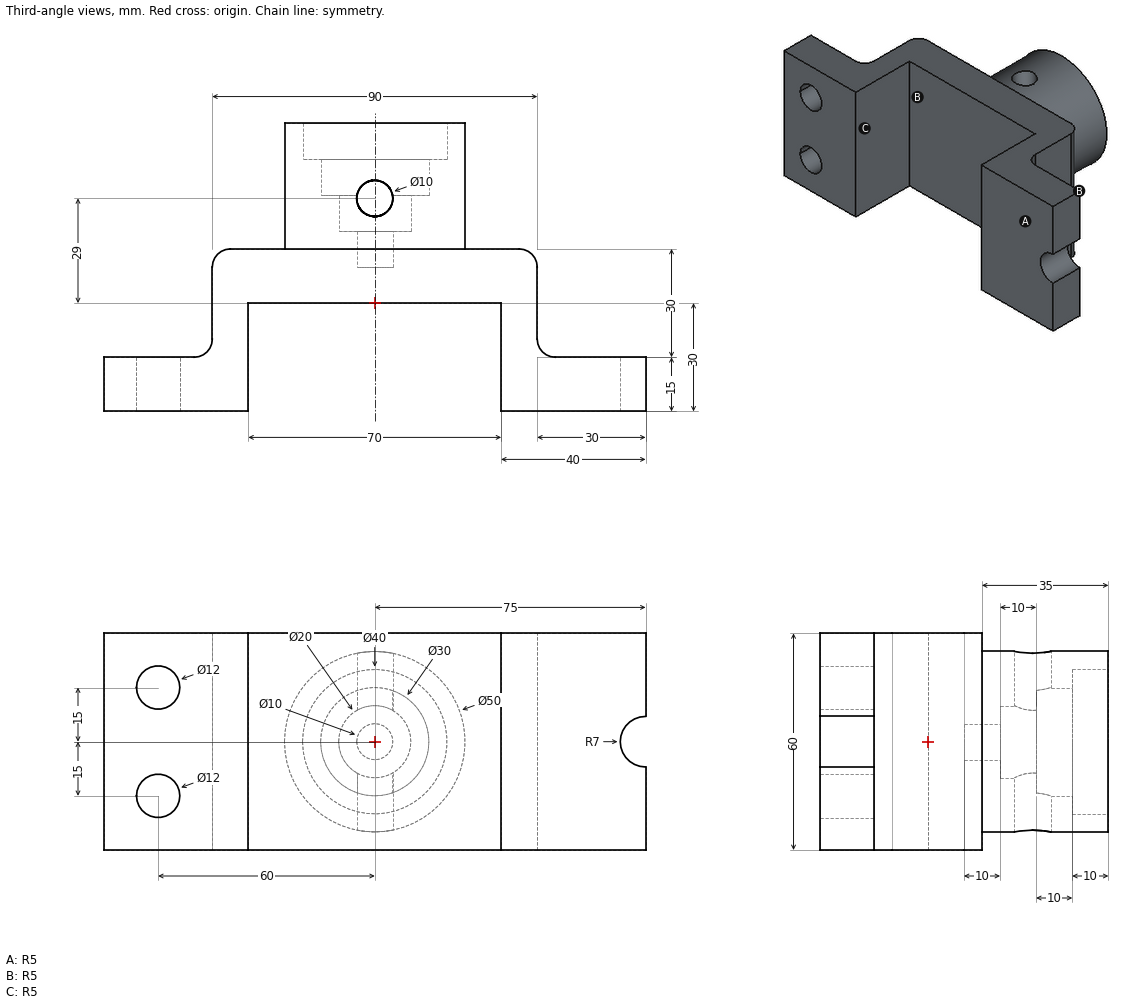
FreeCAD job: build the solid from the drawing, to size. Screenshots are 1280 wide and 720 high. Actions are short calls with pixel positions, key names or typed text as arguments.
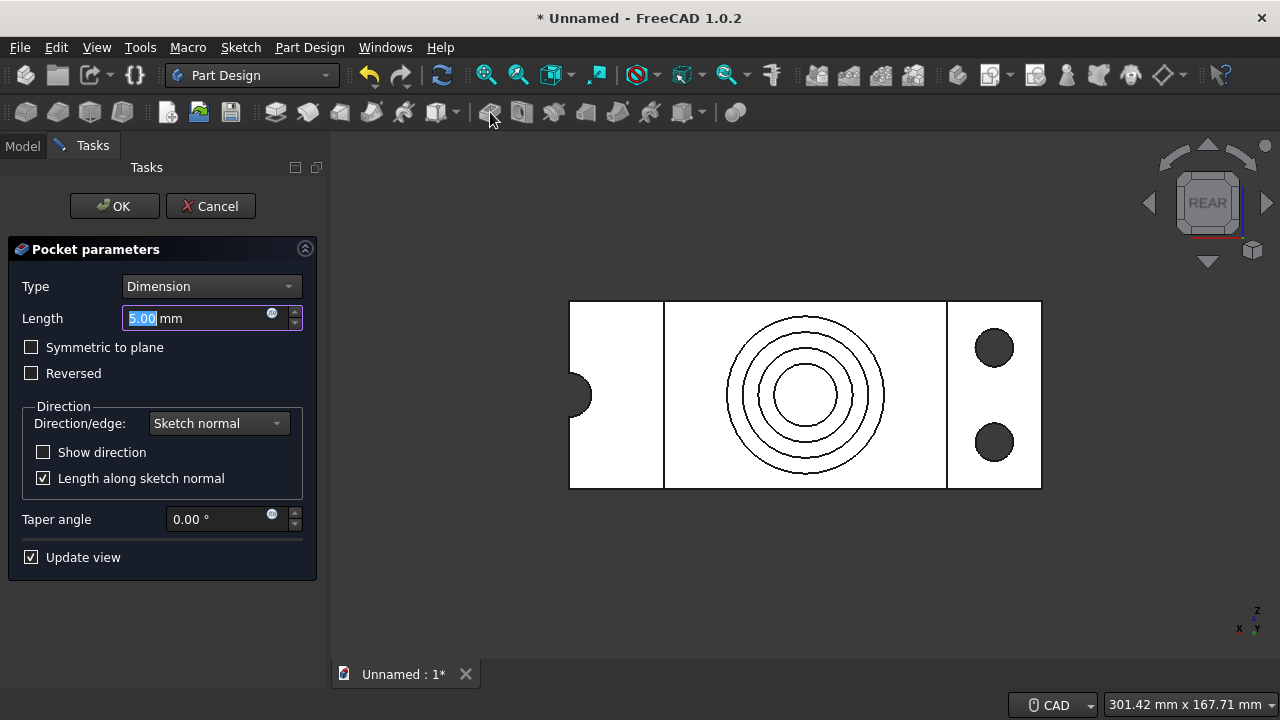
text(10)
key(Tab)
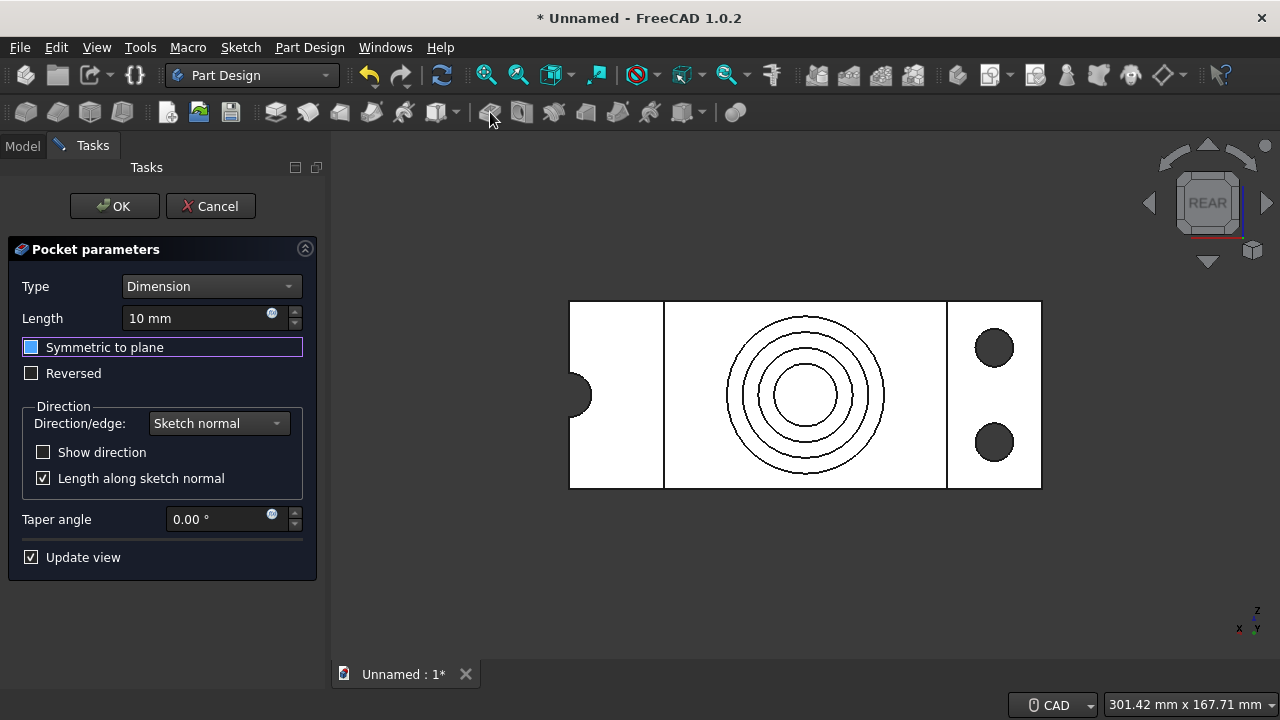
click(115, 206)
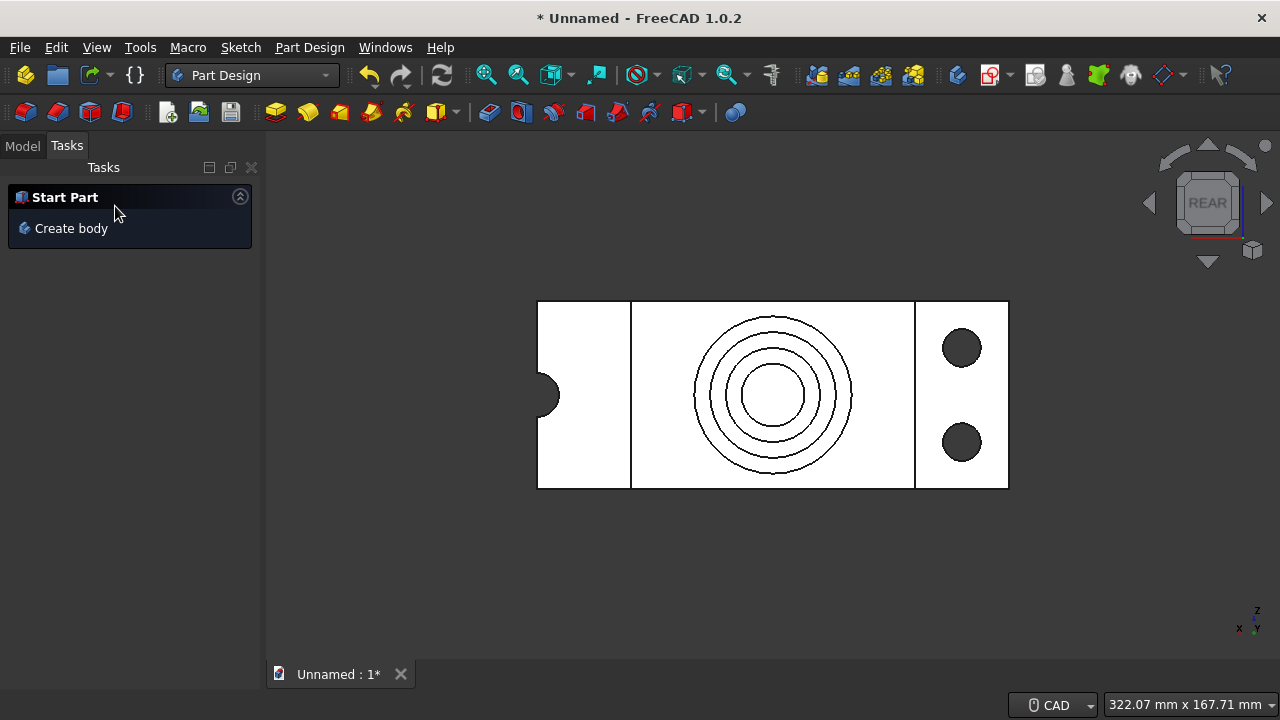
click(773, 394)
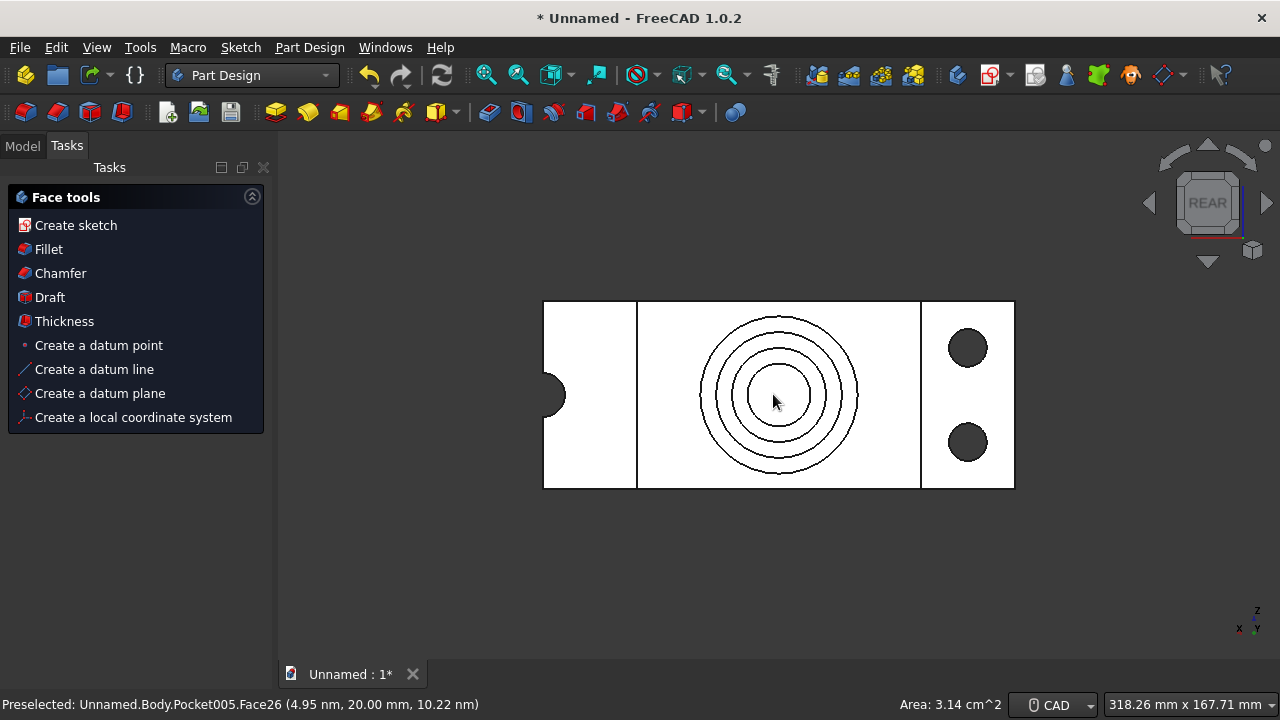
click(990, 76)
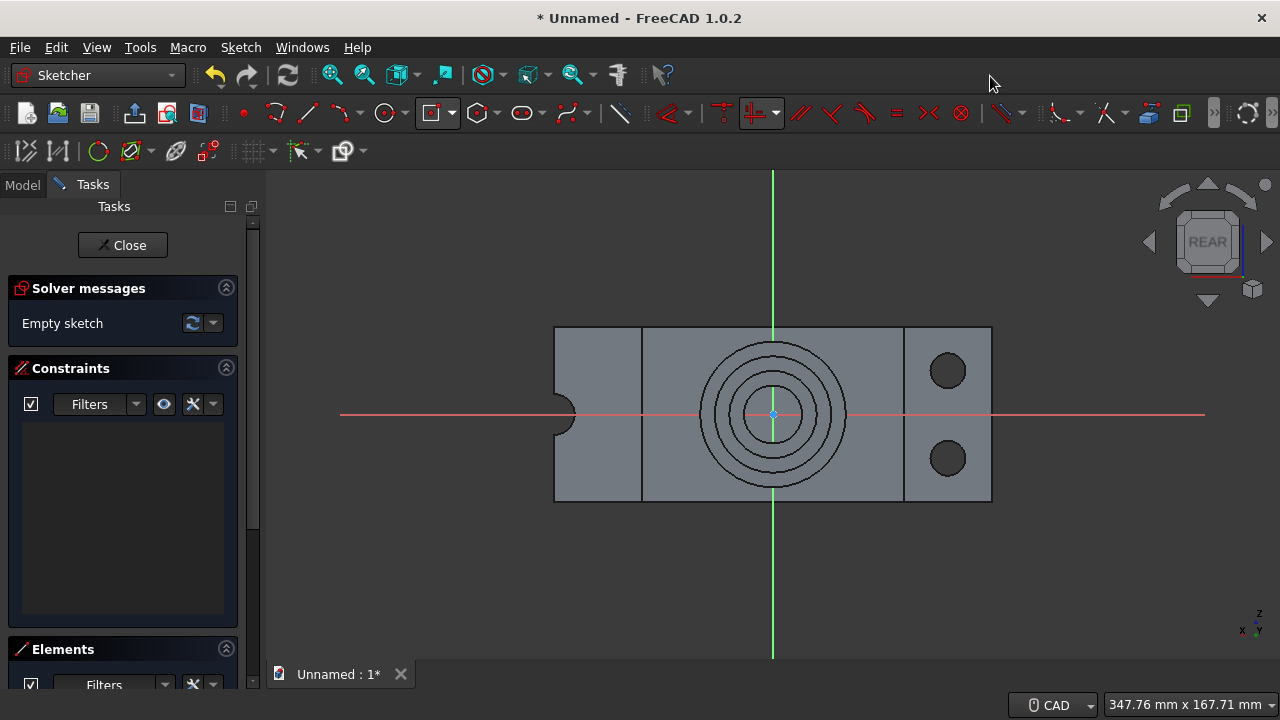
click(200, 114)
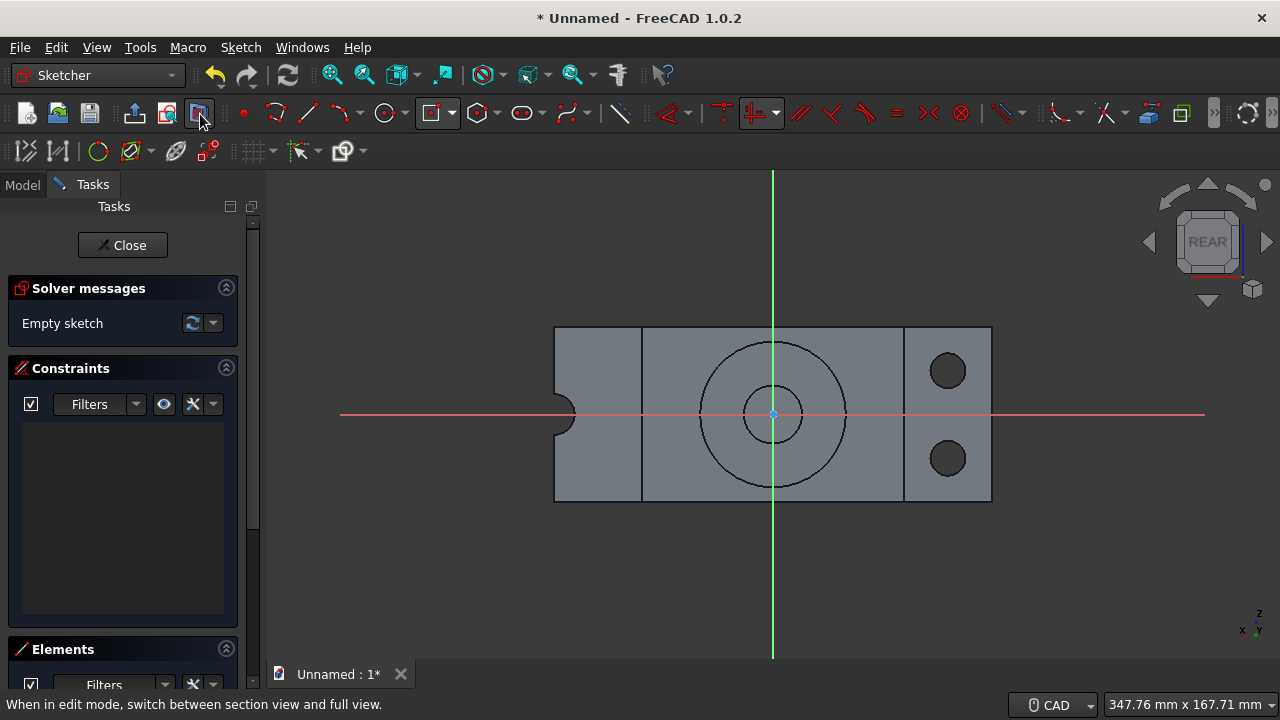
scroll(780, 415, up, 12)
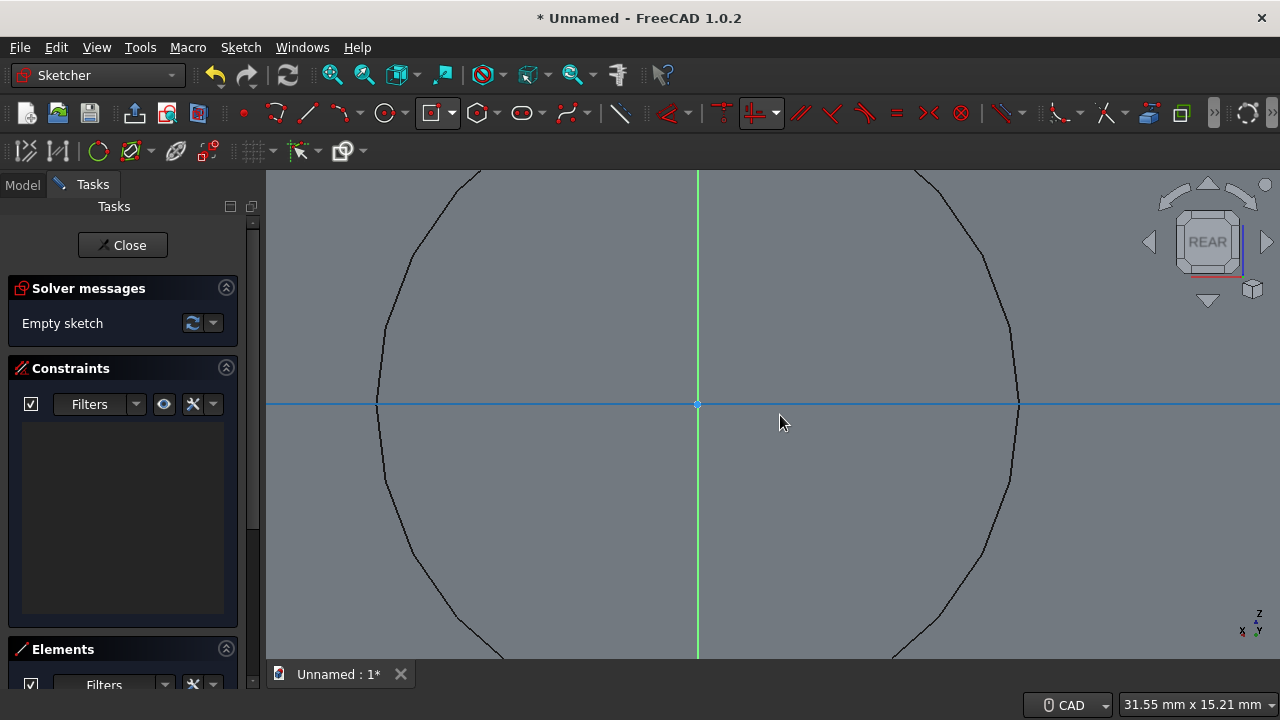
click(386, 114)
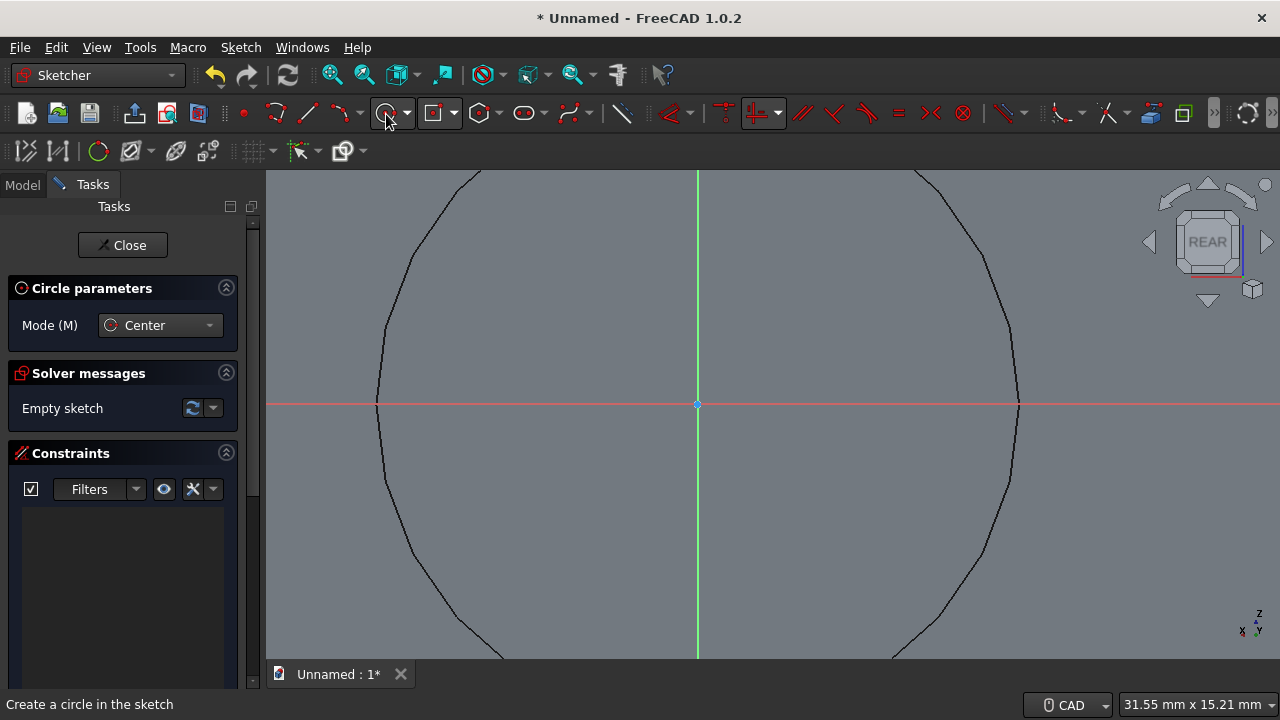
click(698, 404)
click(811, 291)
key(Escape)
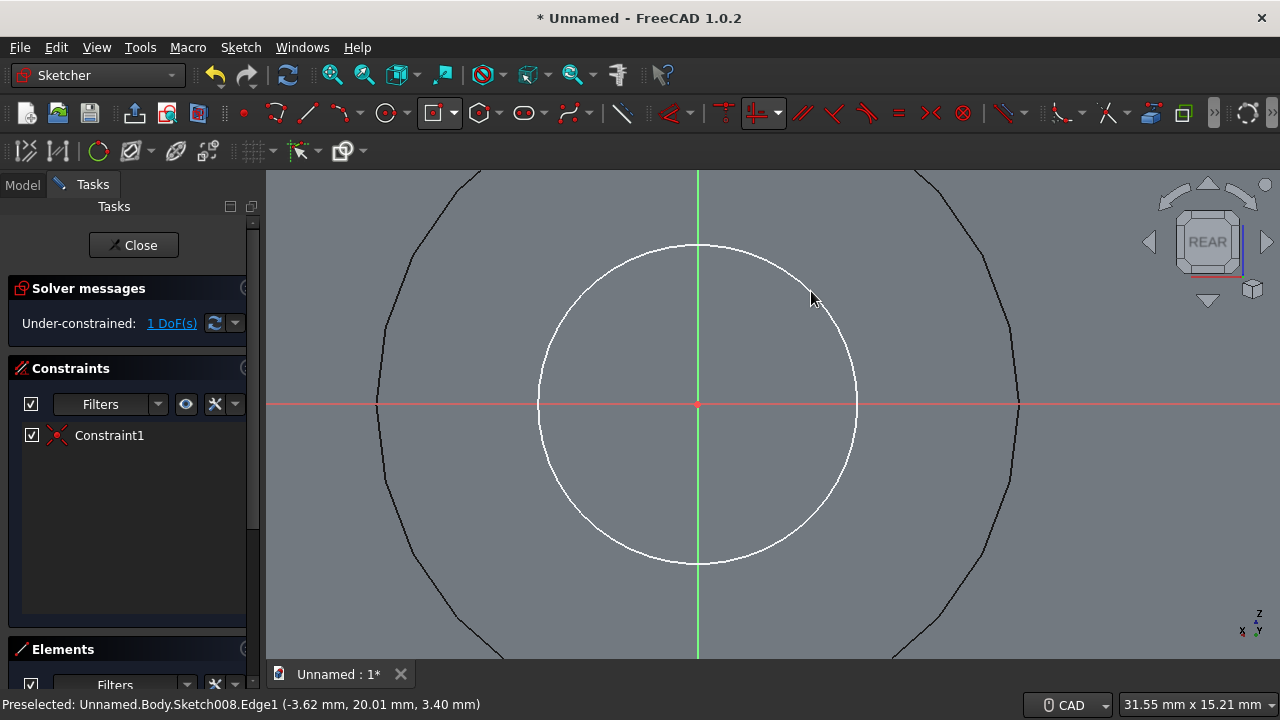
key(d)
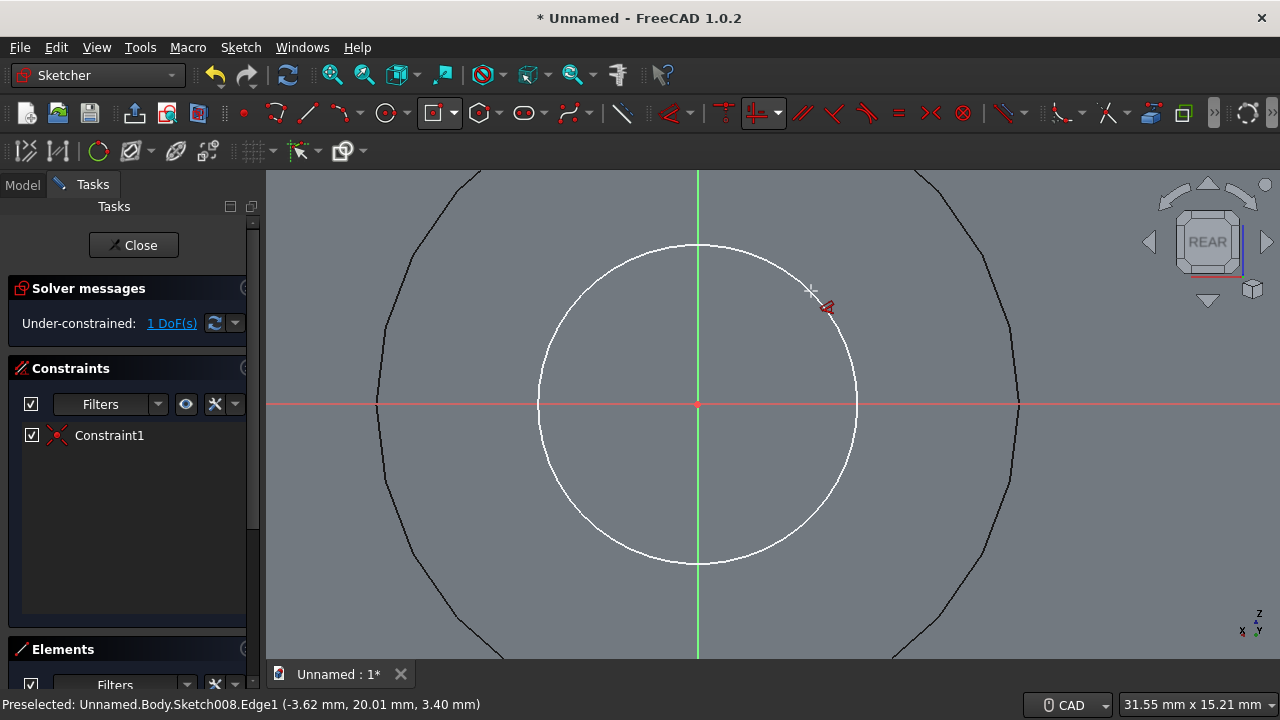
click(810, 291)
click(833, 268)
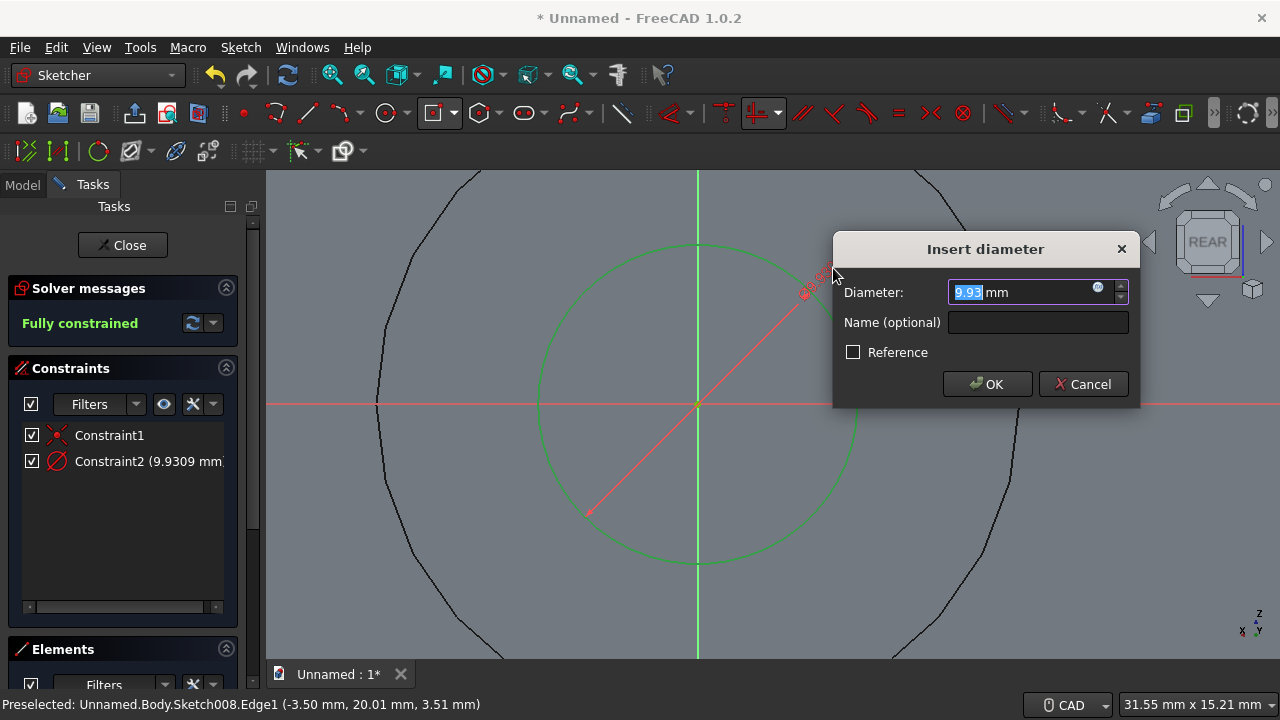
text(10)
key(Return)
key(Escape)